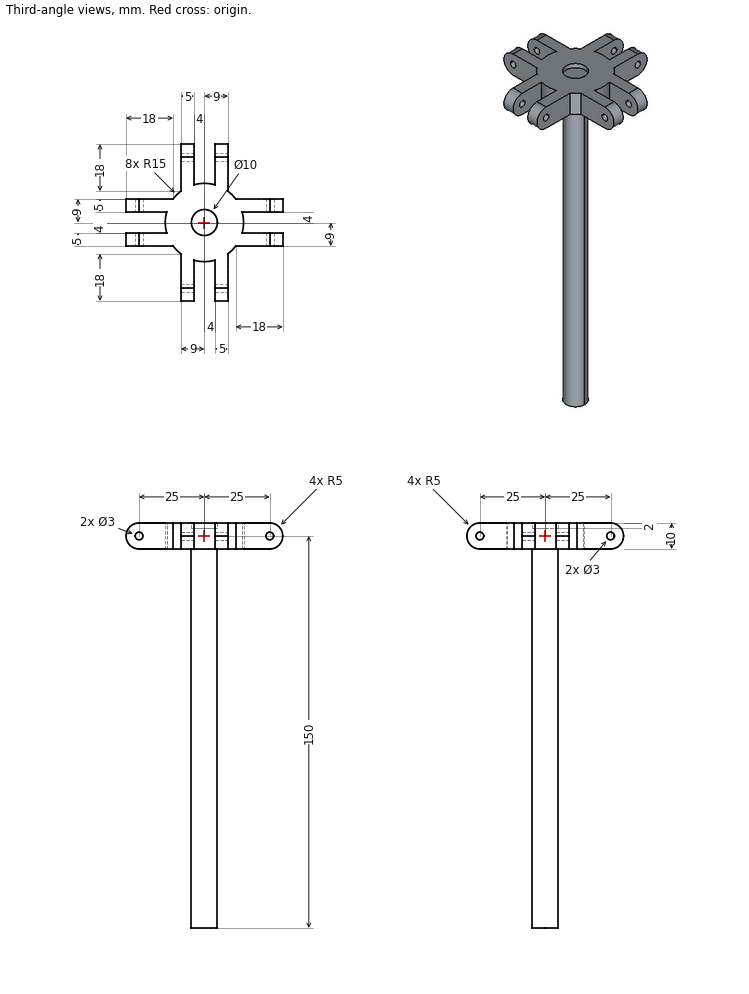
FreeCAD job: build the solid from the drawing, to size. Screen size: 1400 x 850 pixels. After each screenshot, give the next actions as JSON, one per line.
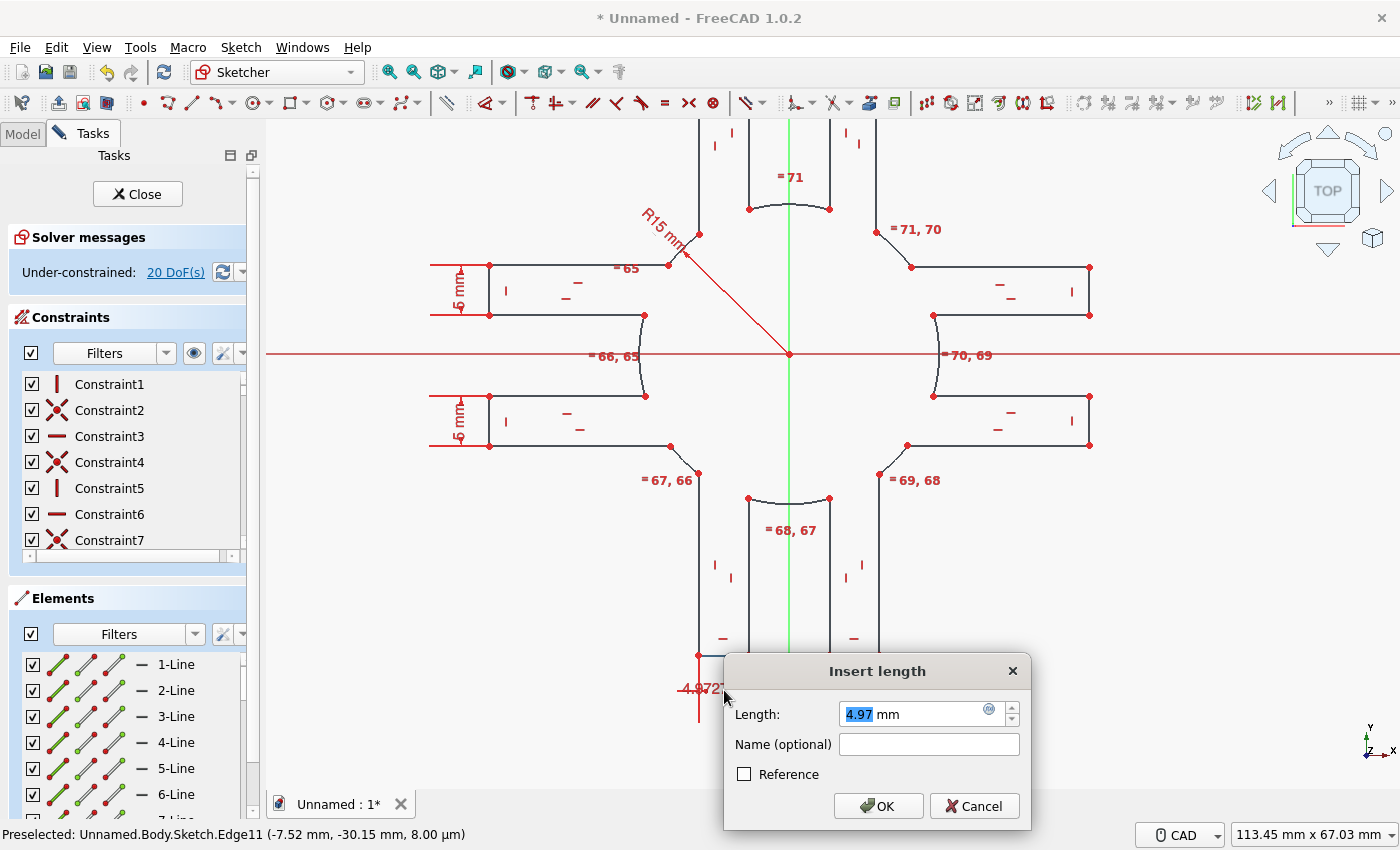
{"action": "type", "text": "5"}
{"action": "key", "text": "Return"}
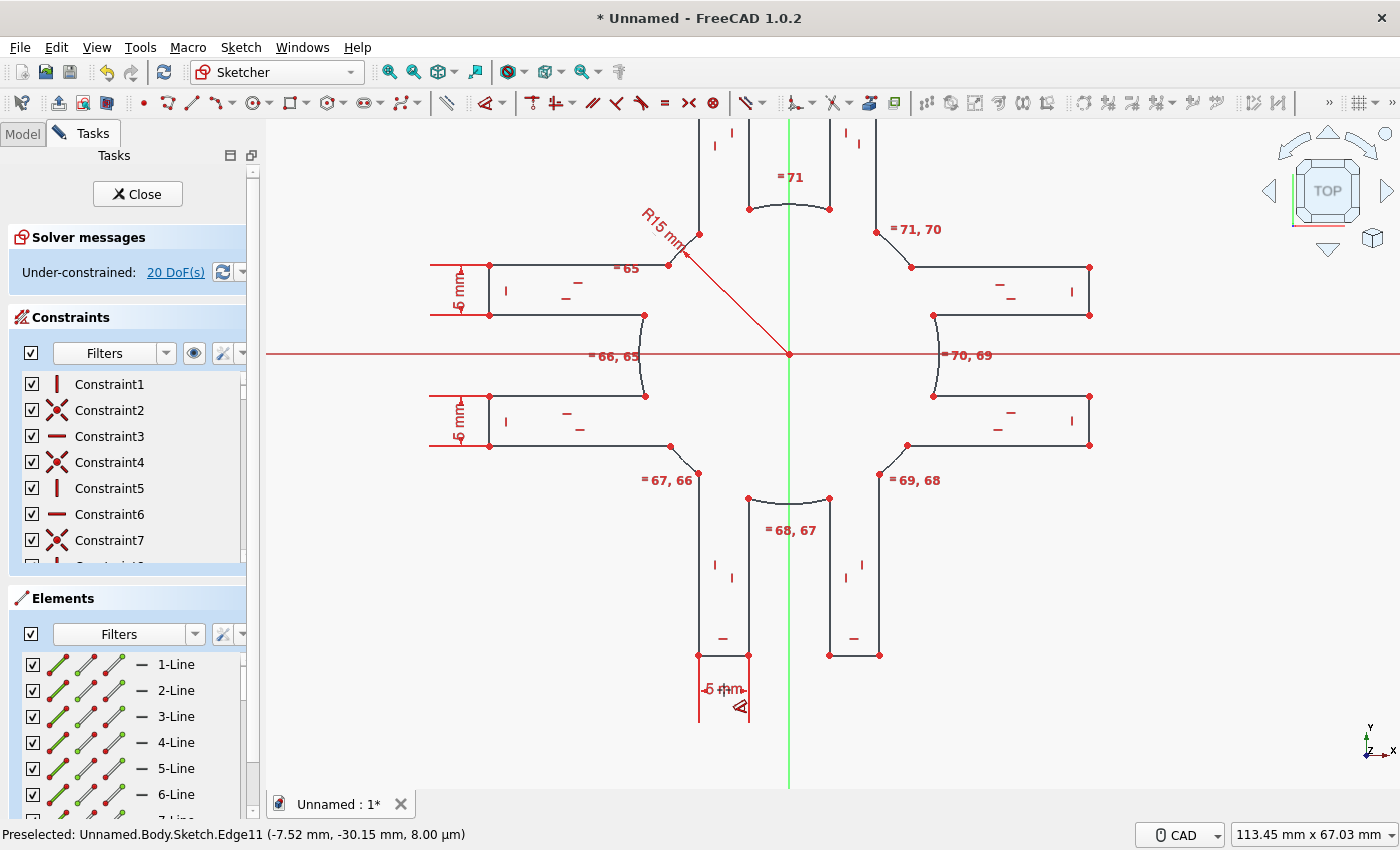
{"action": "left_click", "coordinate": [845, 656]}
{"action": "left_click", "coordinate": [854, 690]}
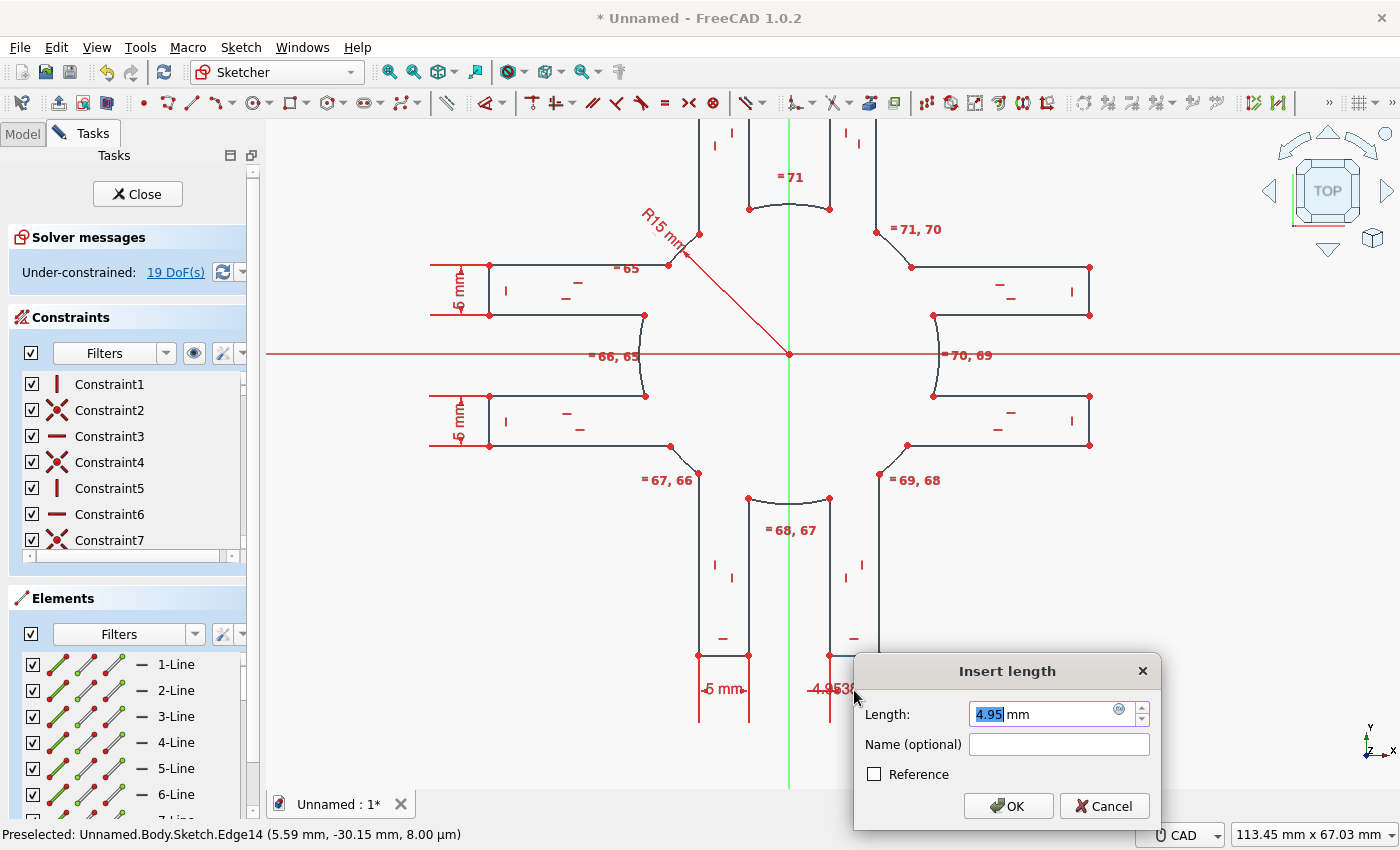
{"action": "type", "text": "5"}
{"action": "key", "text": "Return"}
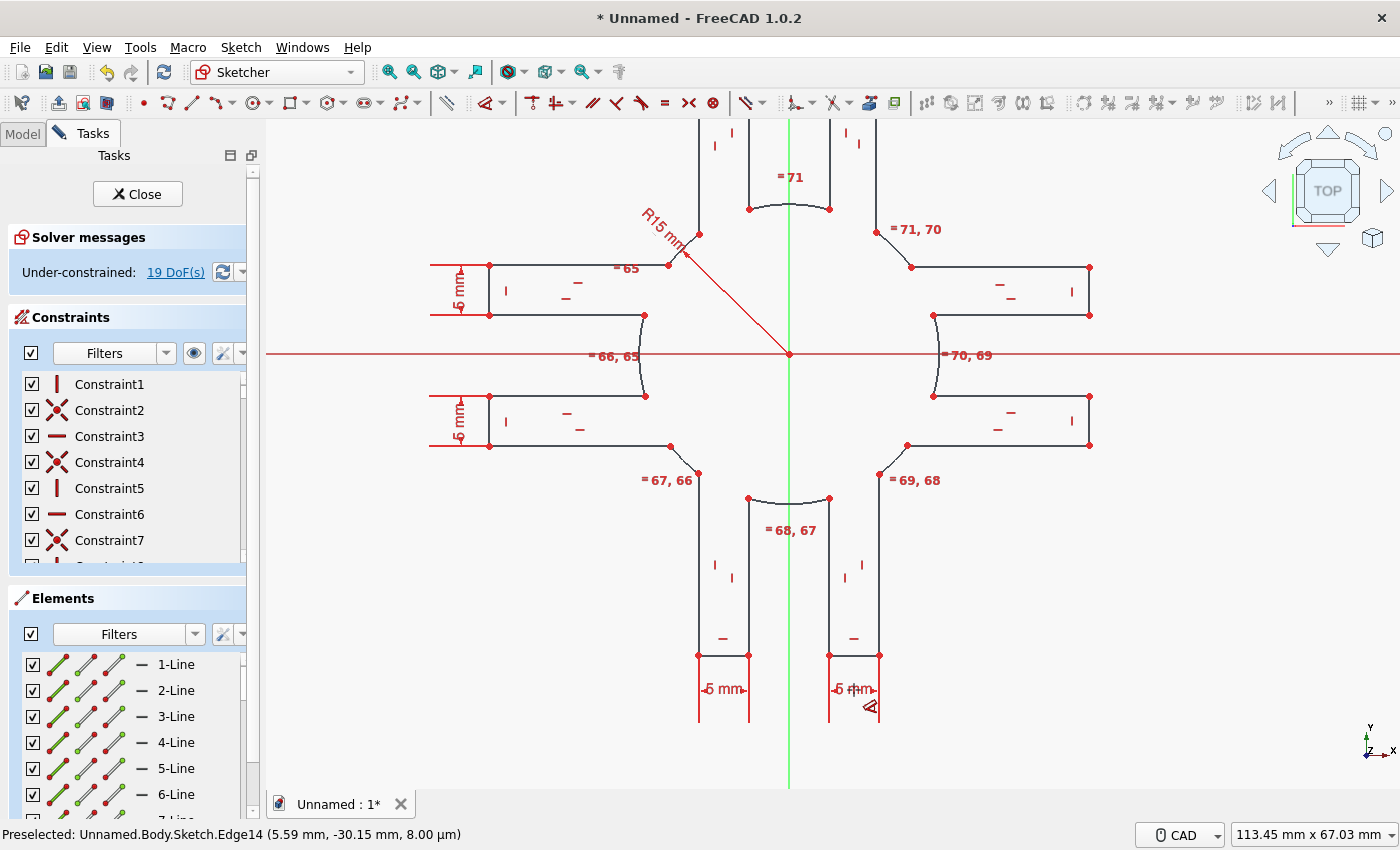
{"action": "left_click", "coordinate": [1089, 431]}
{"action": "left_click", "coordinate": [1123, 421]}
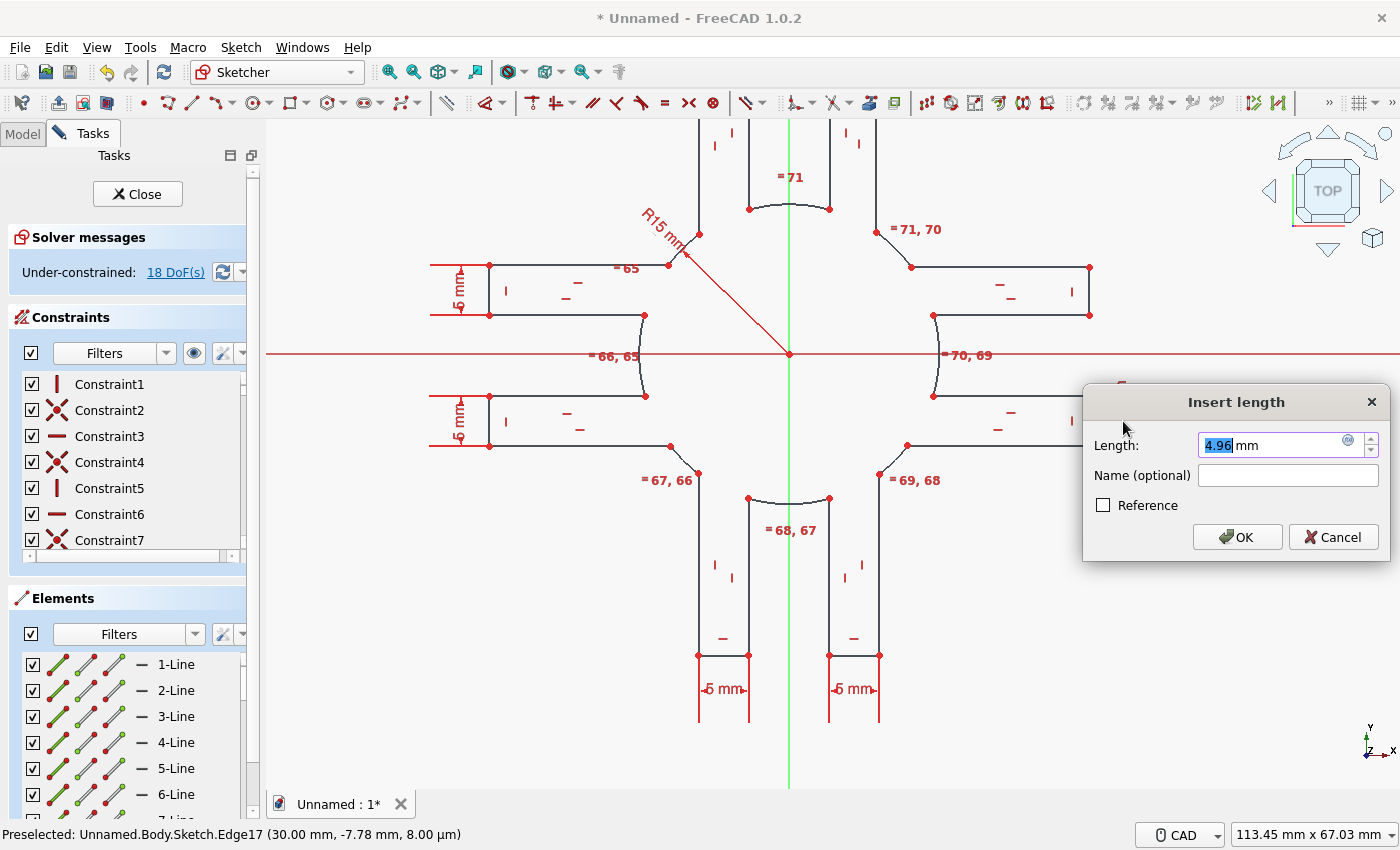
{"action": "type", "text": "5"}
{"action": "key", "text": "Return"}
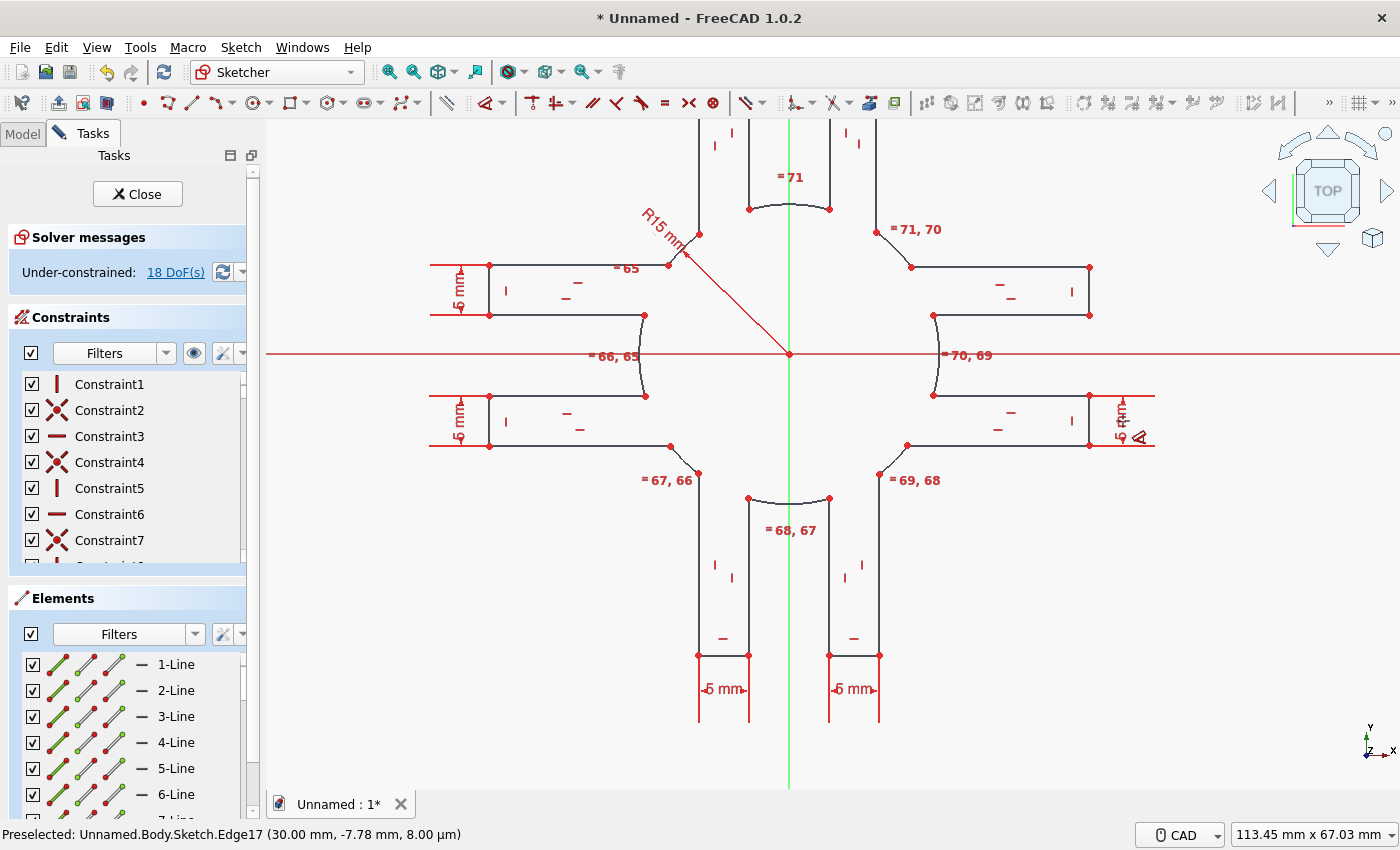
{"action": "left_click", "coordinate": [1089, 301]}
{"action": "left_click", "coordinate": [1123, 291]}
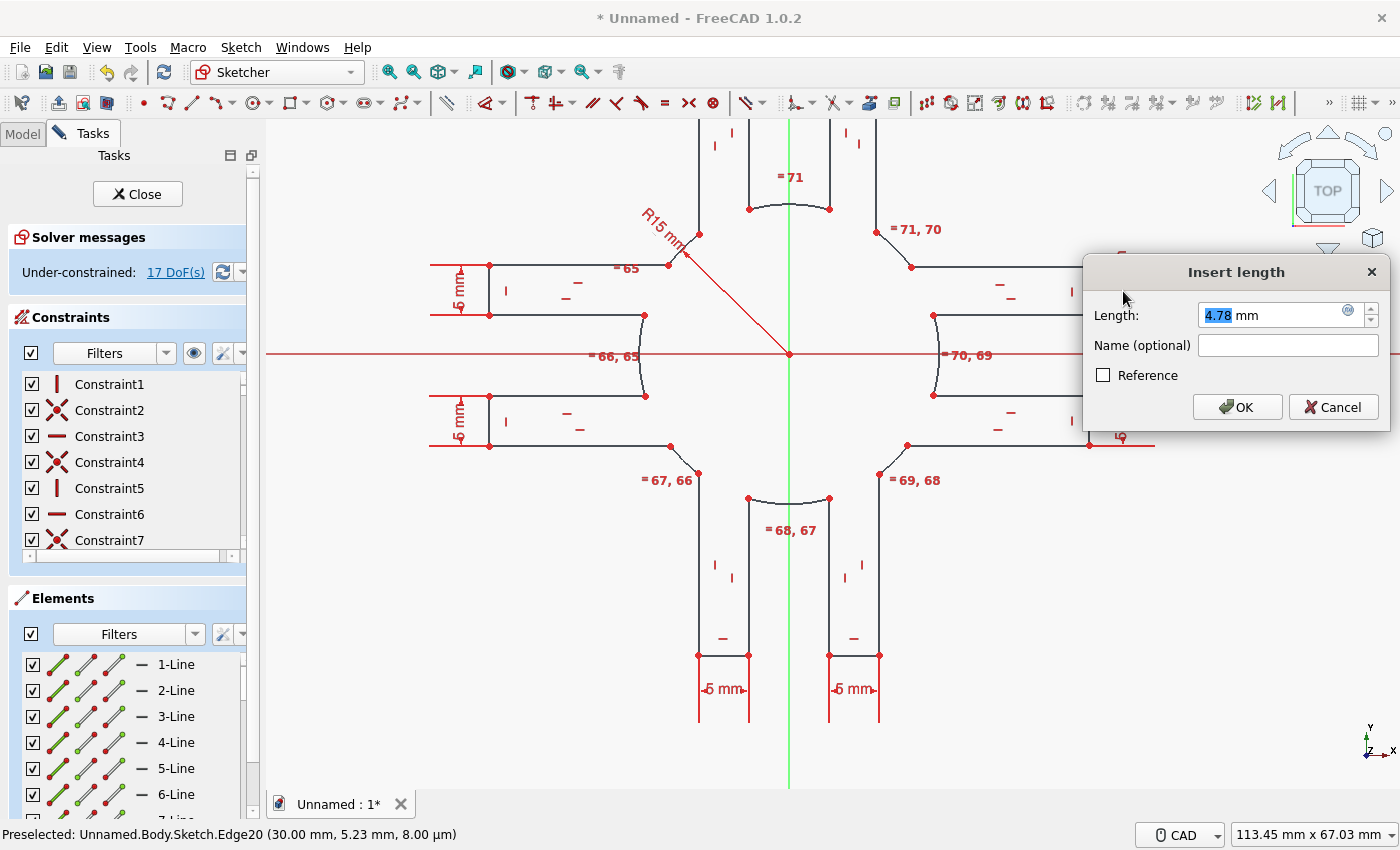
{"action": "type", "text": "5"}
{"action": "key", "text": "Return"}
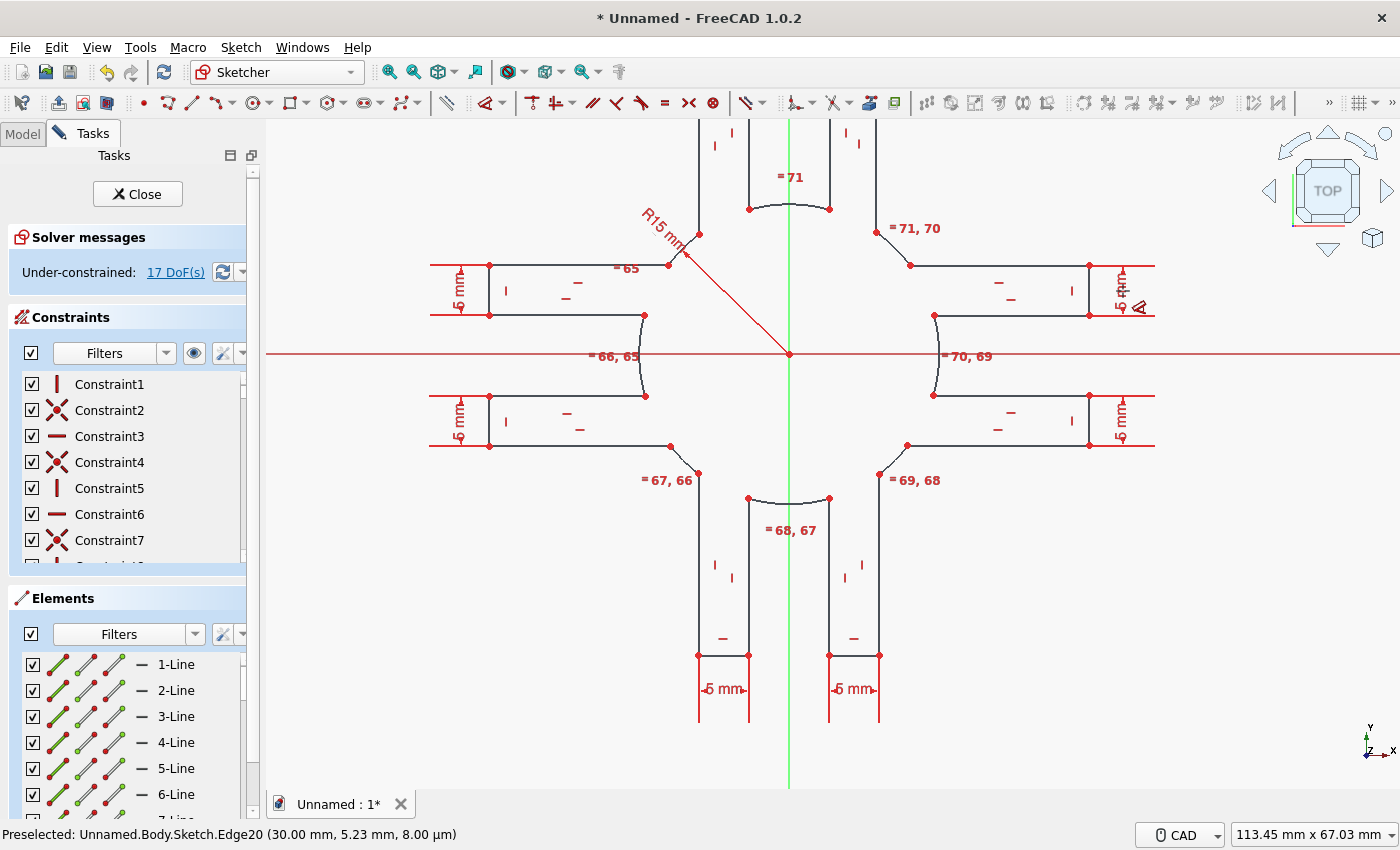
{"action": "scroll", "coordinate": [714, 657], "scroll_direction": "down", "scroll_amount": 2}